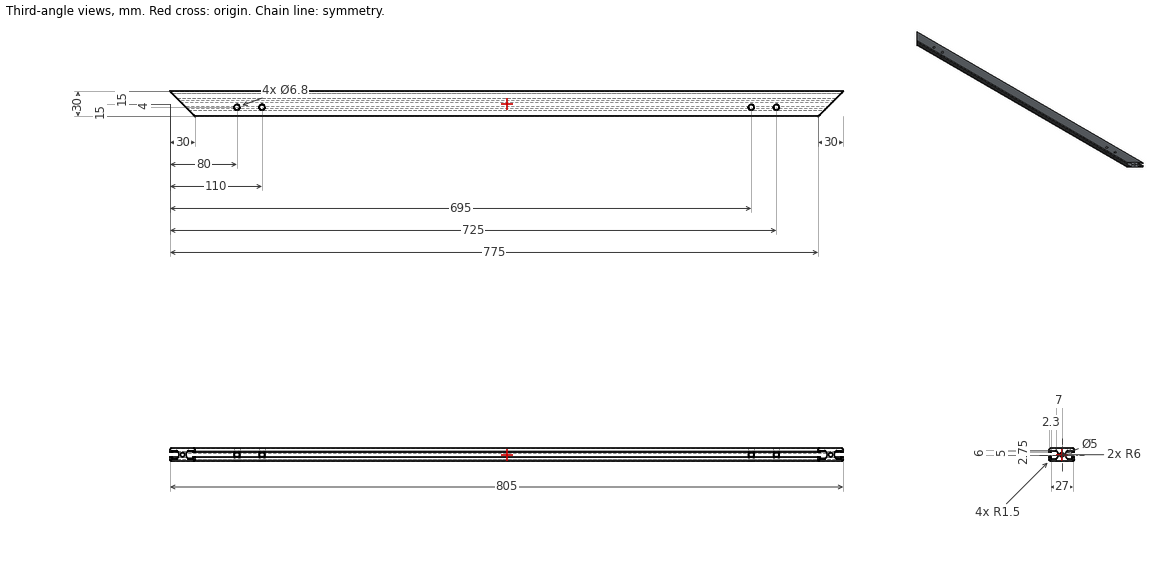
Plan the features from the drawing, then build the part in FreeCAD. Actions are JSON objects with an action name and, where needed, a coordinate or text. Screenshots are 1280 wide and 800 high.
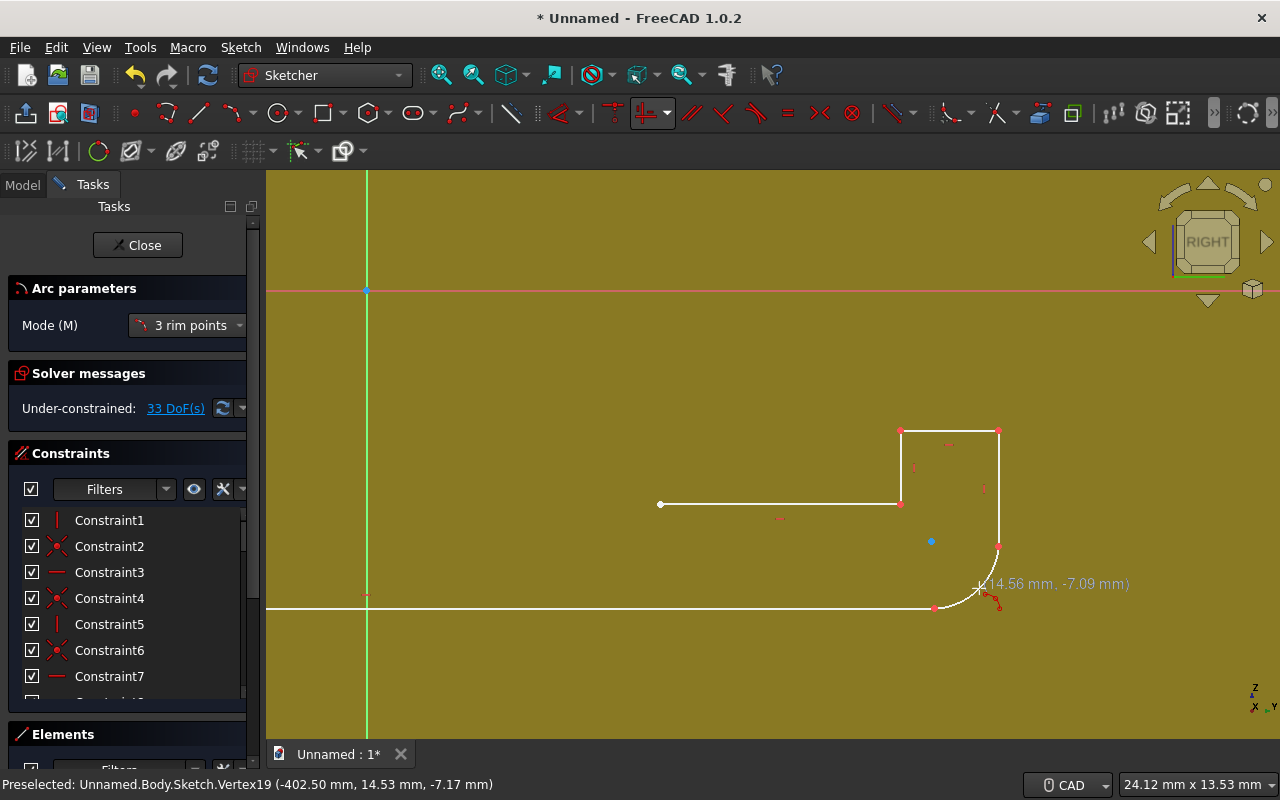
{"action": "left_click", "coordinate": [660, 504]}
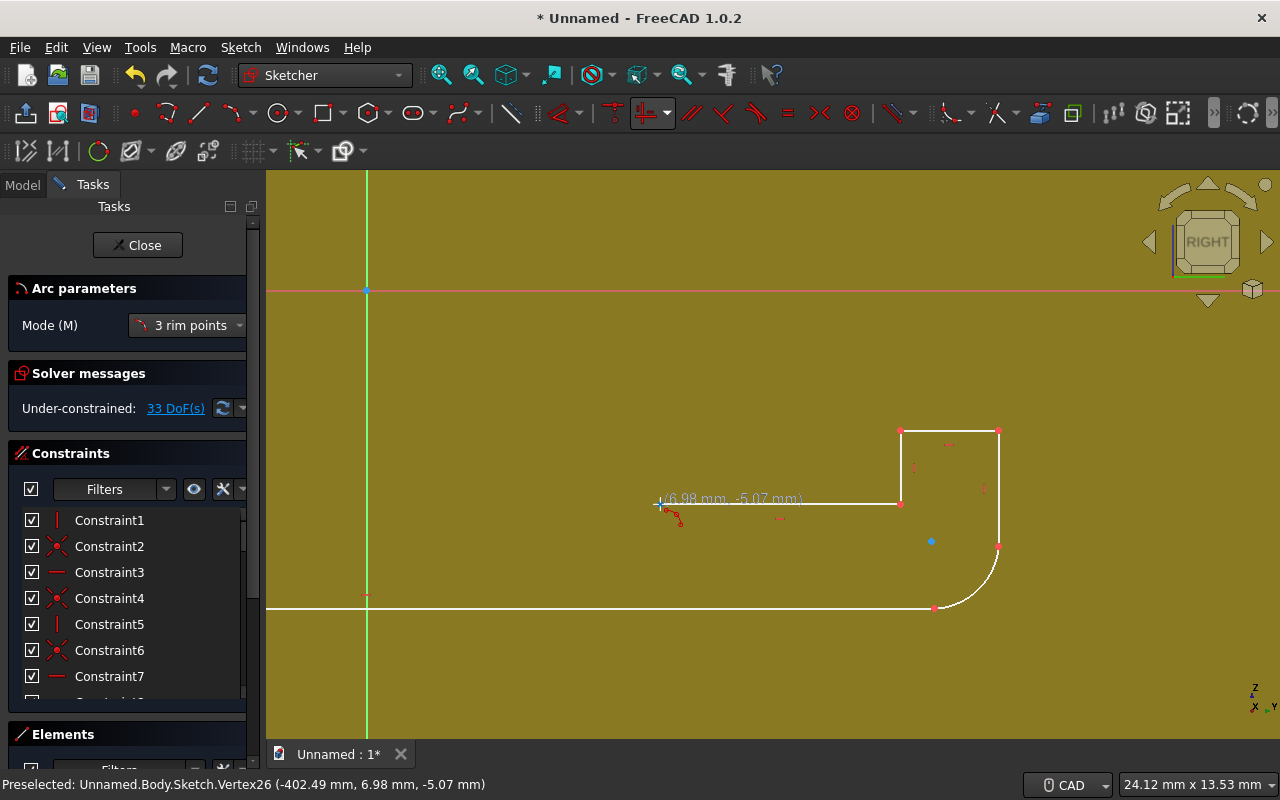
{"action": "scroll", "coordinate": [980, 588], "scroll_direction": "down", "scroll_amount": 4}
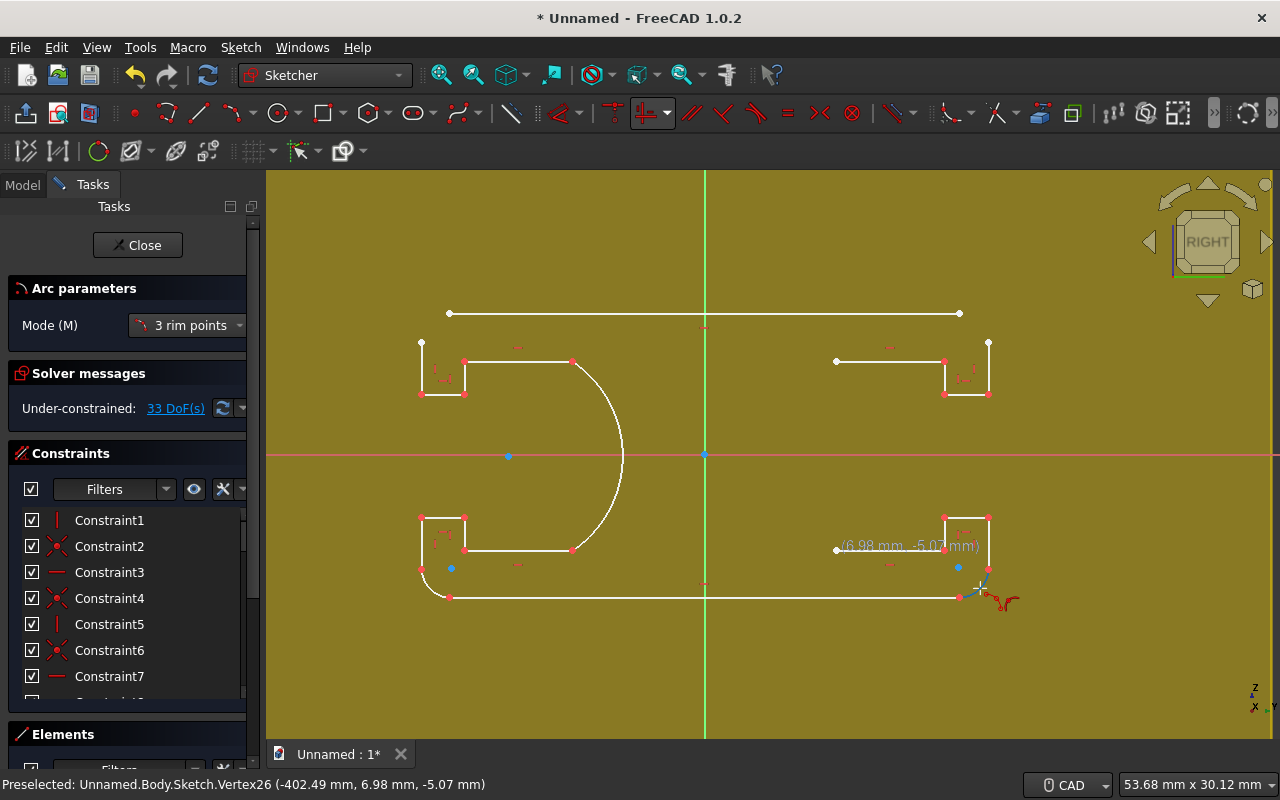
{"action": "left_click", "coordinate": [837, 362]}
{"action": "left_click", "coordinate": [789, 433]}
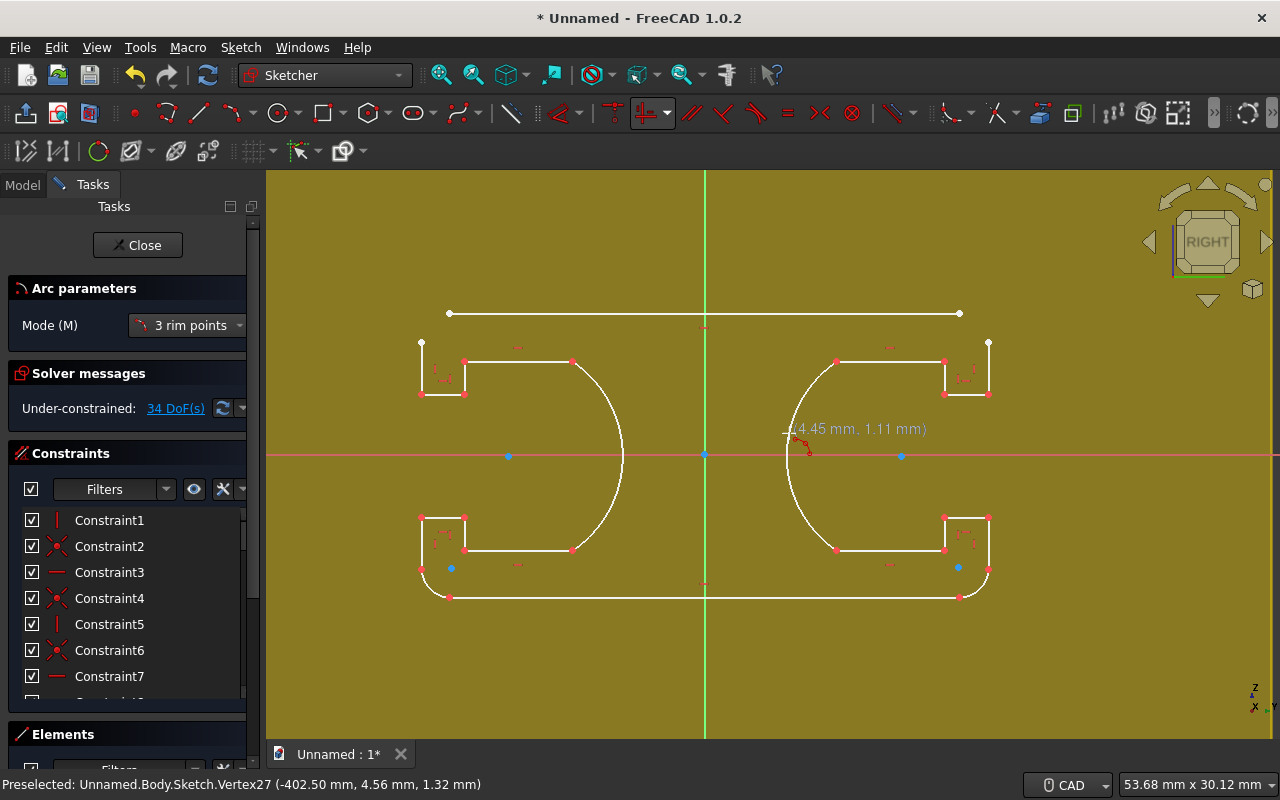
{"action": "left_click", "coordinate": [989, 343]}
{"action": "left_click", "coordinate": [960, 314]}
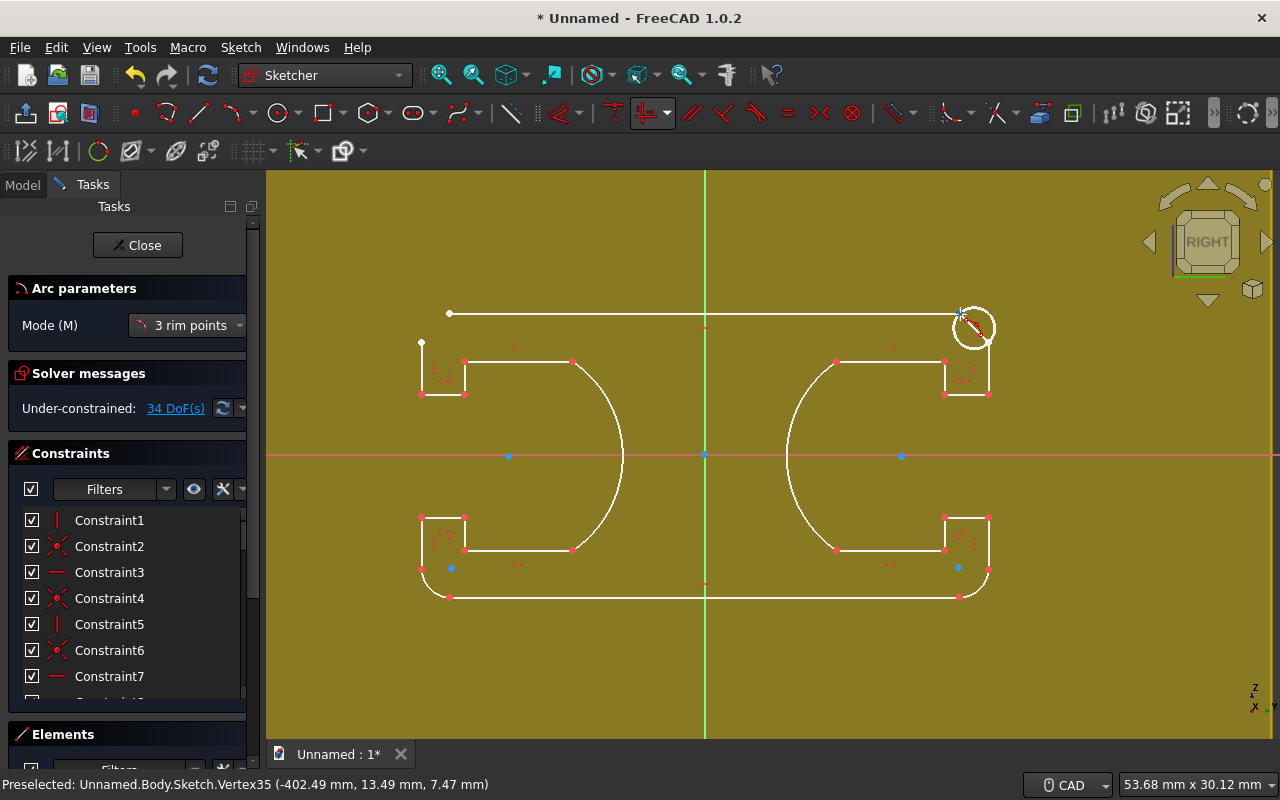
{"action": "scroll", "coordinate": [980, 322], "scroll_direction": "up", "scroll_amount": 4}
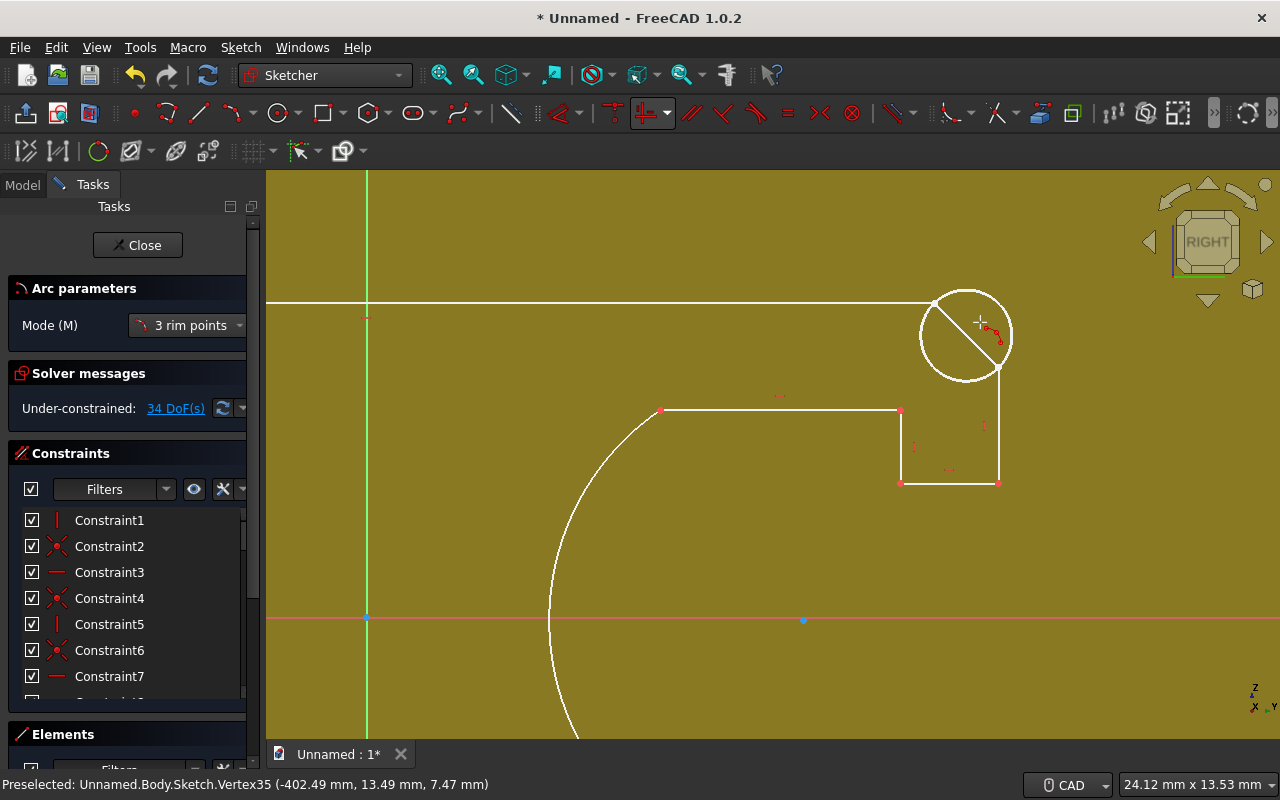
{"action": "left_click", "coordinate": [979, 321]}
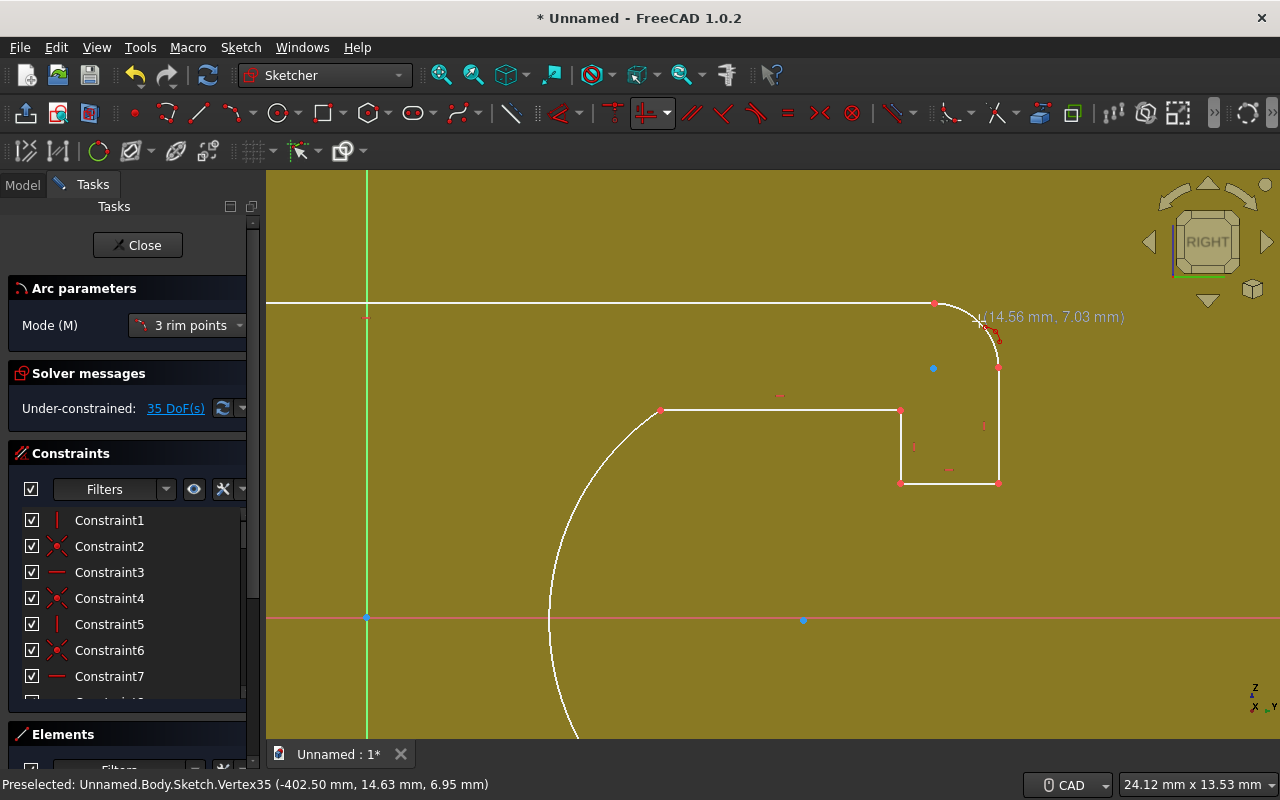
{"action": "scroll", "coordinate": [980, 321], "scroll_direction": "down", "scroll_amount": 4}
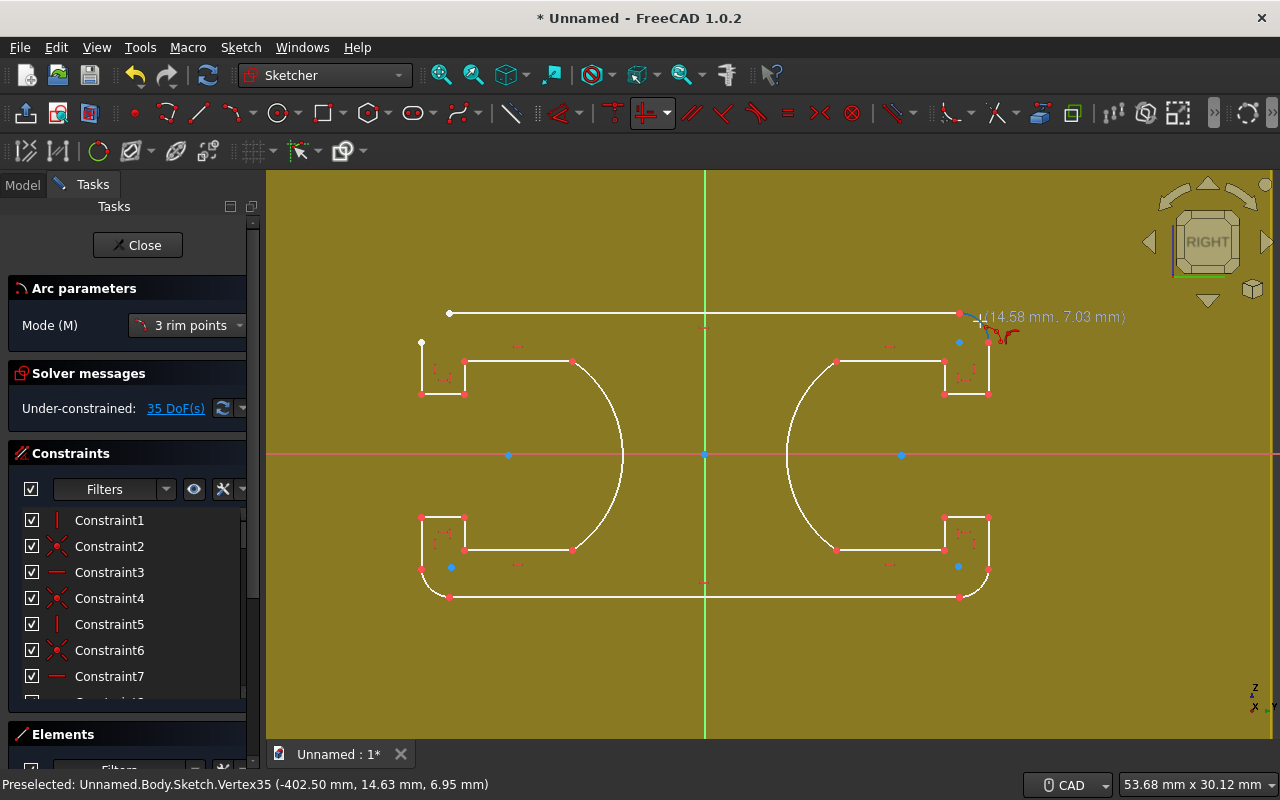
{"action": "left_click", "coordinate": [450, 313]}
{"action": "left_click", "coordinate": [422, 342]}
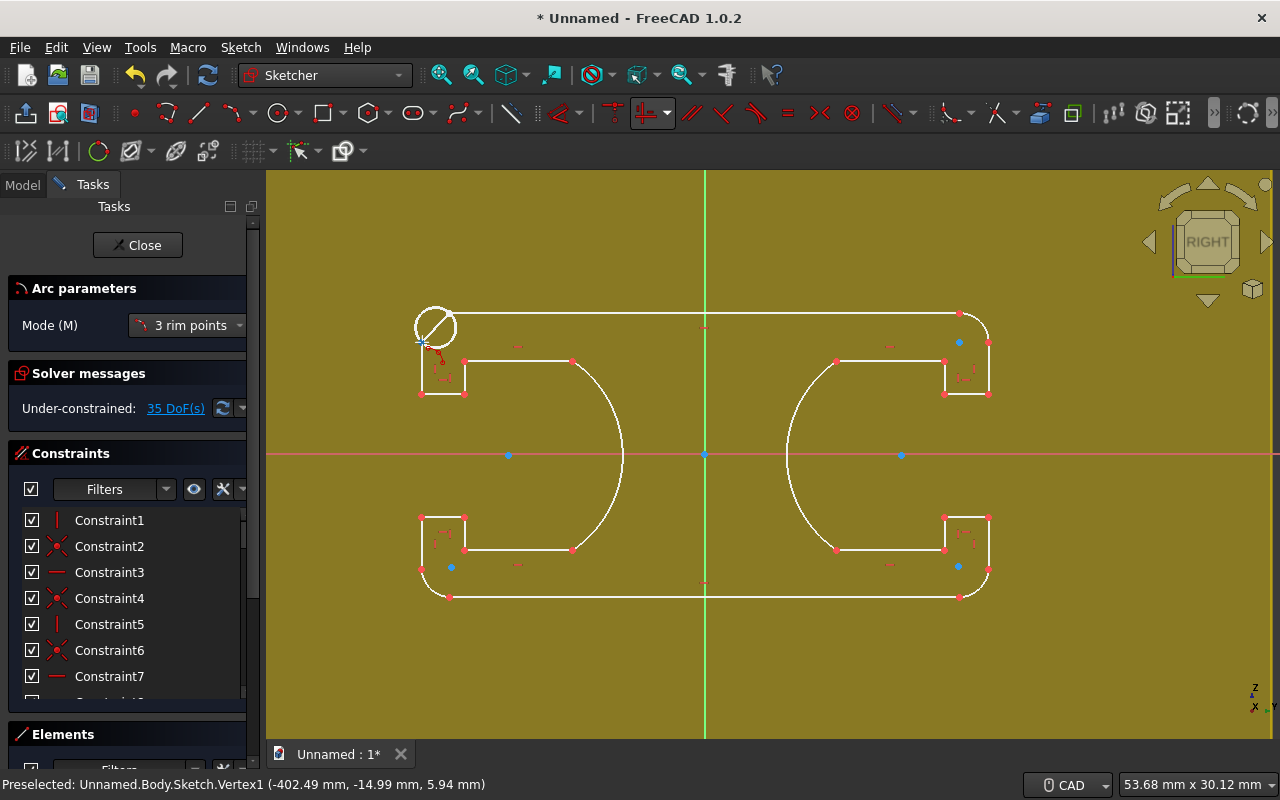
{"action": "scroll", "coordinate": [430, 321], "scroll_direction": "up", "scroll_amount": 4}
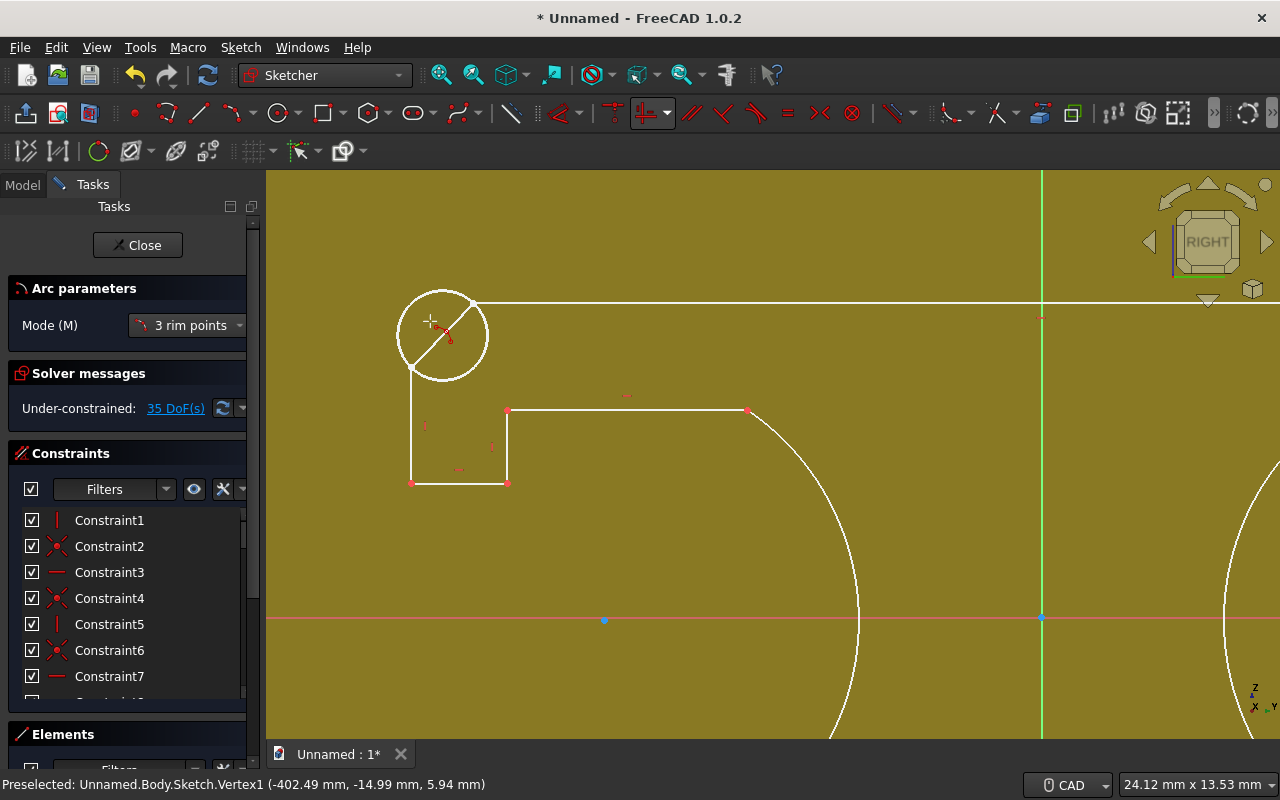
{"action": "left_click", "coordinate": [429, 321]}